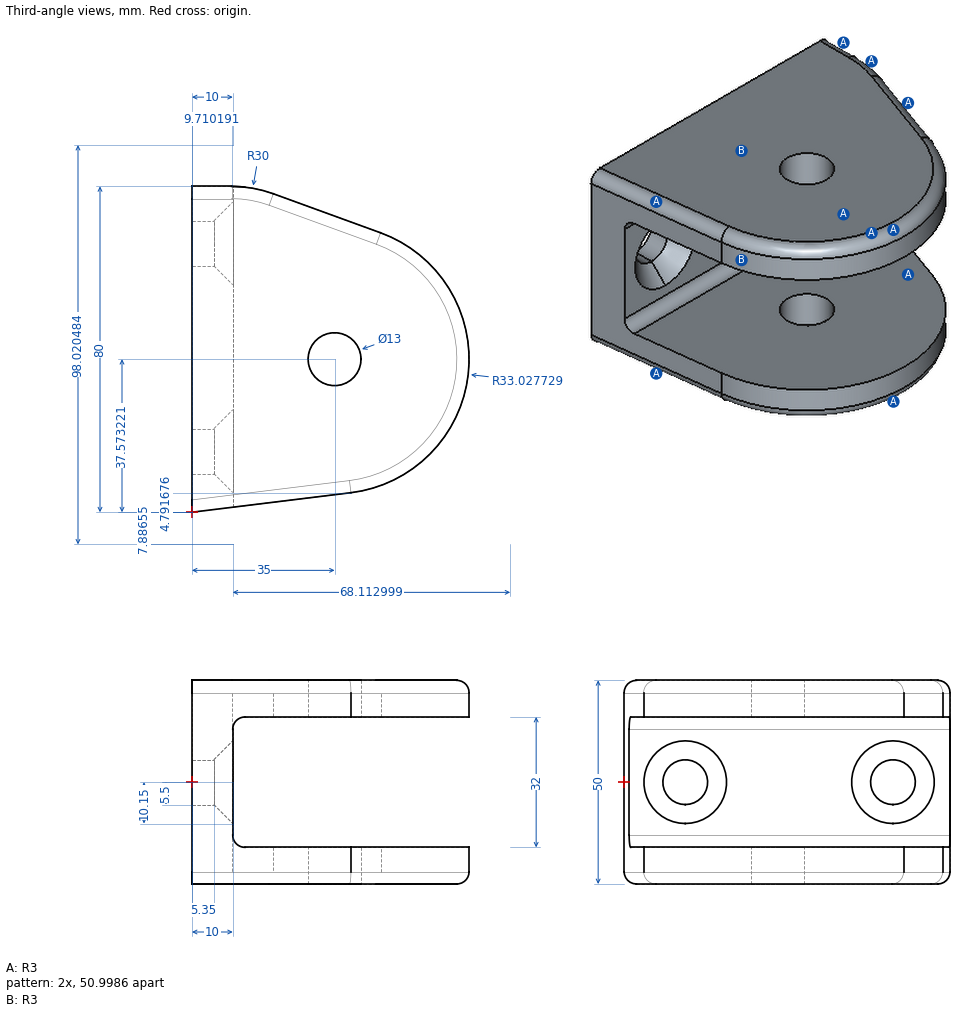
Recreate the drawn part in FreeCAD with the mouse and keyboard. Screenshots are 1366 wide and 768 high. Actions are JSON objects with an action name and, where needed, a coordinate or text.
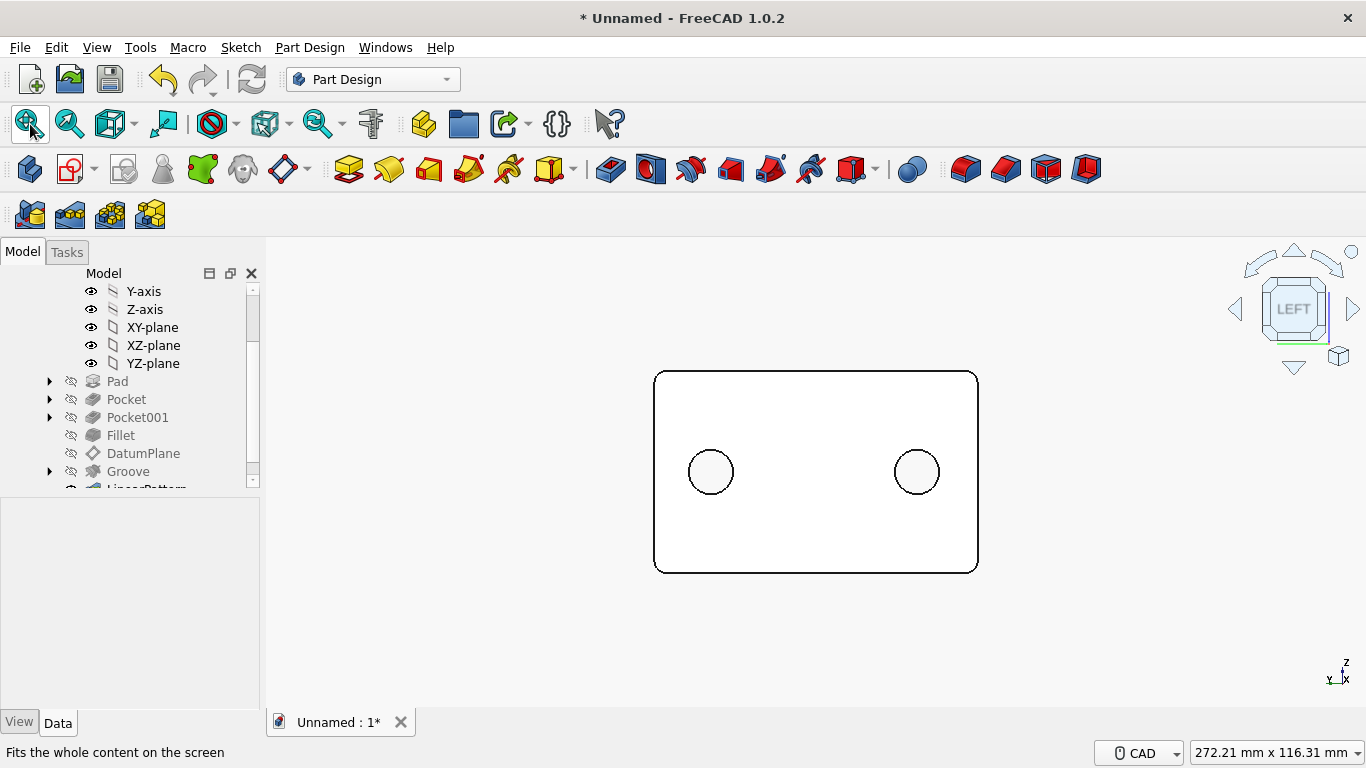
{"action": "key", "text": "v 3"}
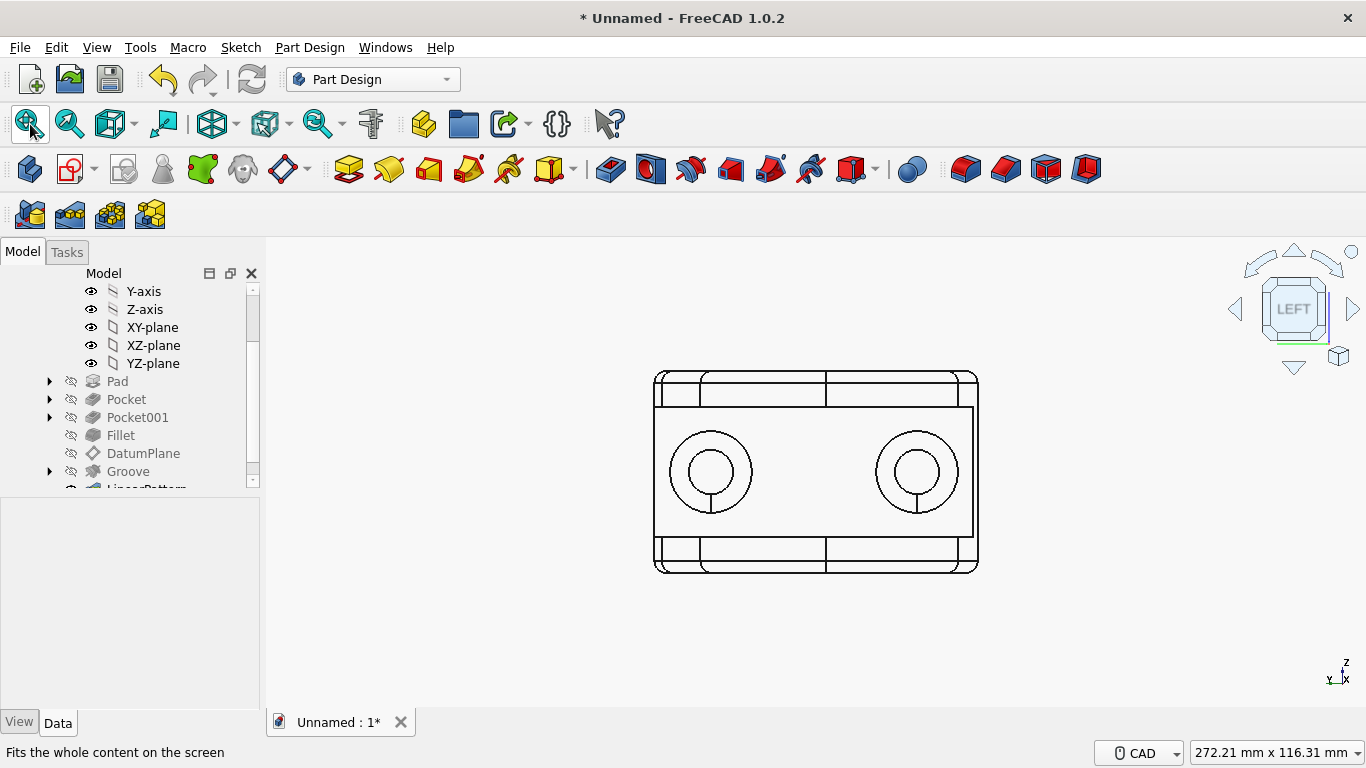
{"action": "key", "text": "0"}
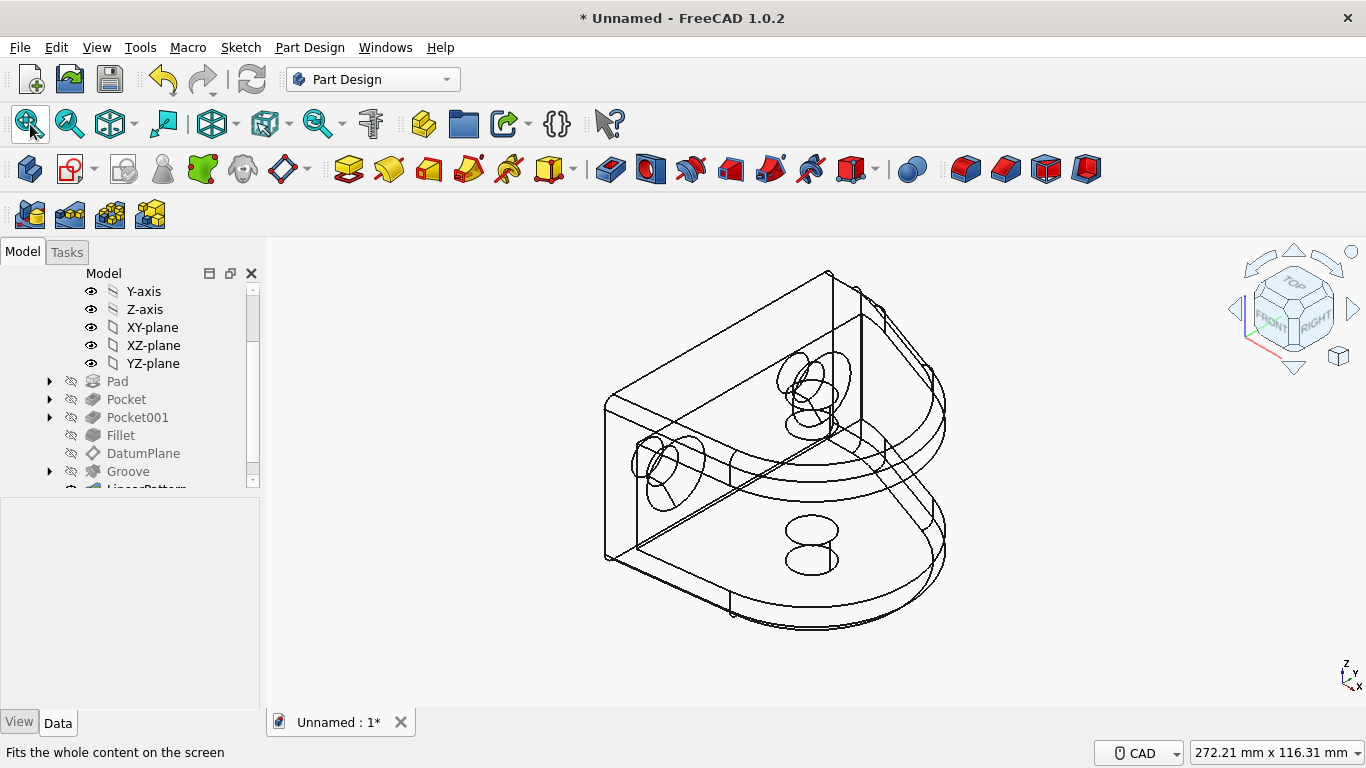
{"action": "left_click", "coordinate": [749, 483]}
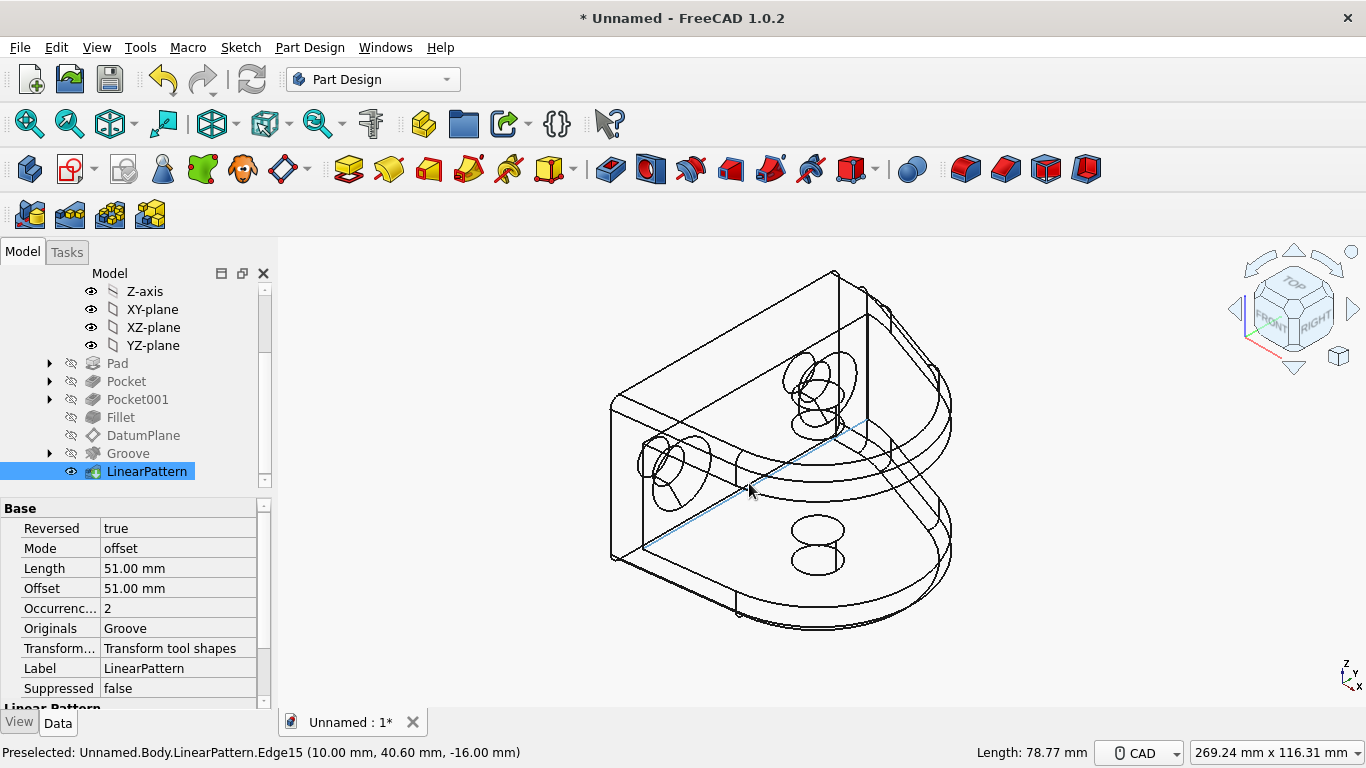
{"action": "left_click", "coordinate": [755, 378], "text": "ctrl"}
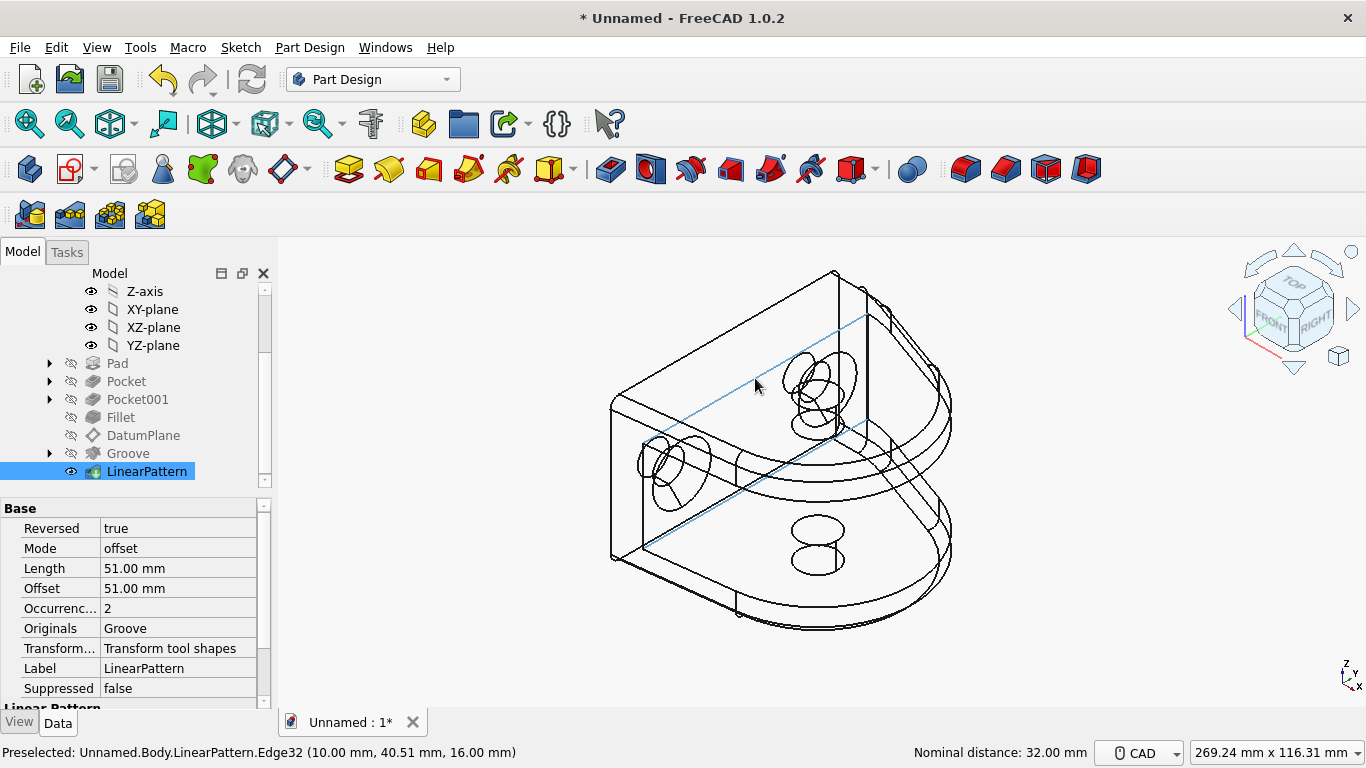
{"action": "key", "text": "v 1"}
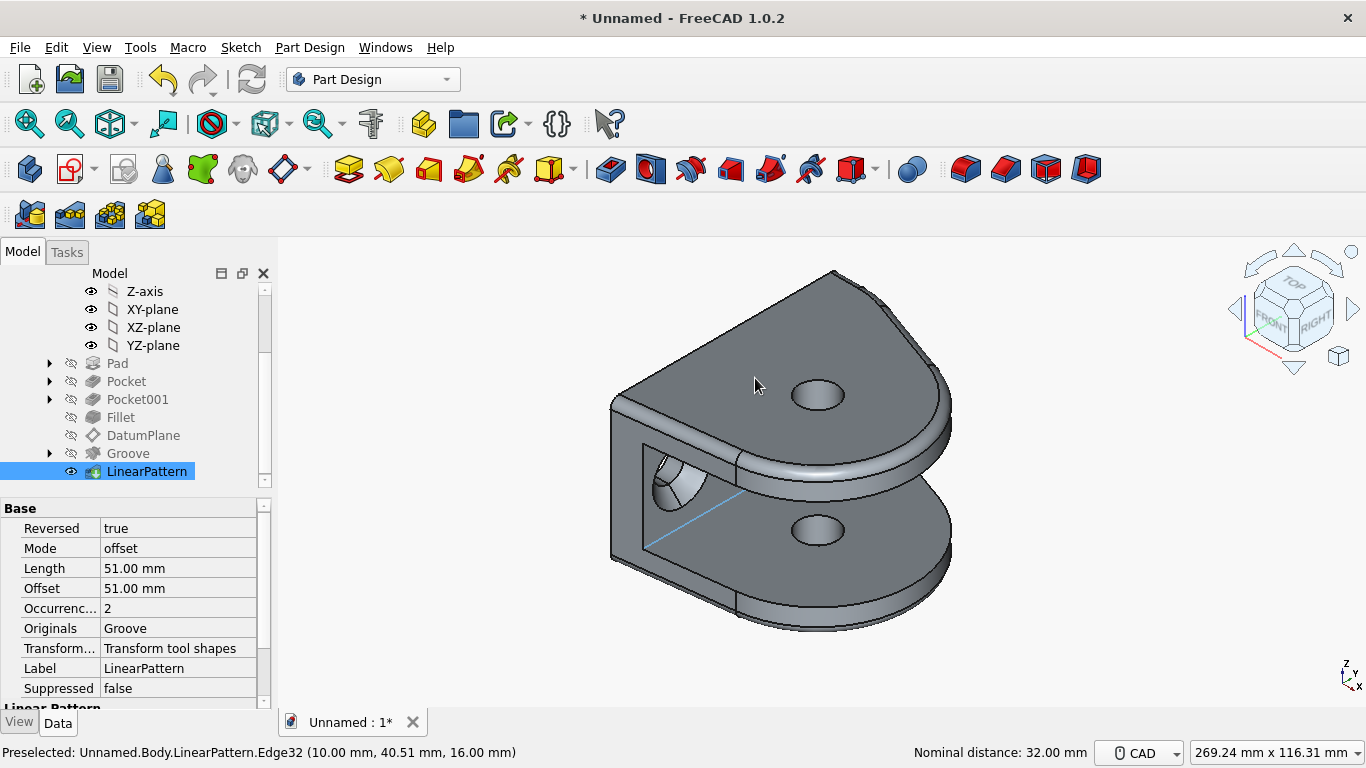
{"action": "left_click", "coordinate": [966, 170]}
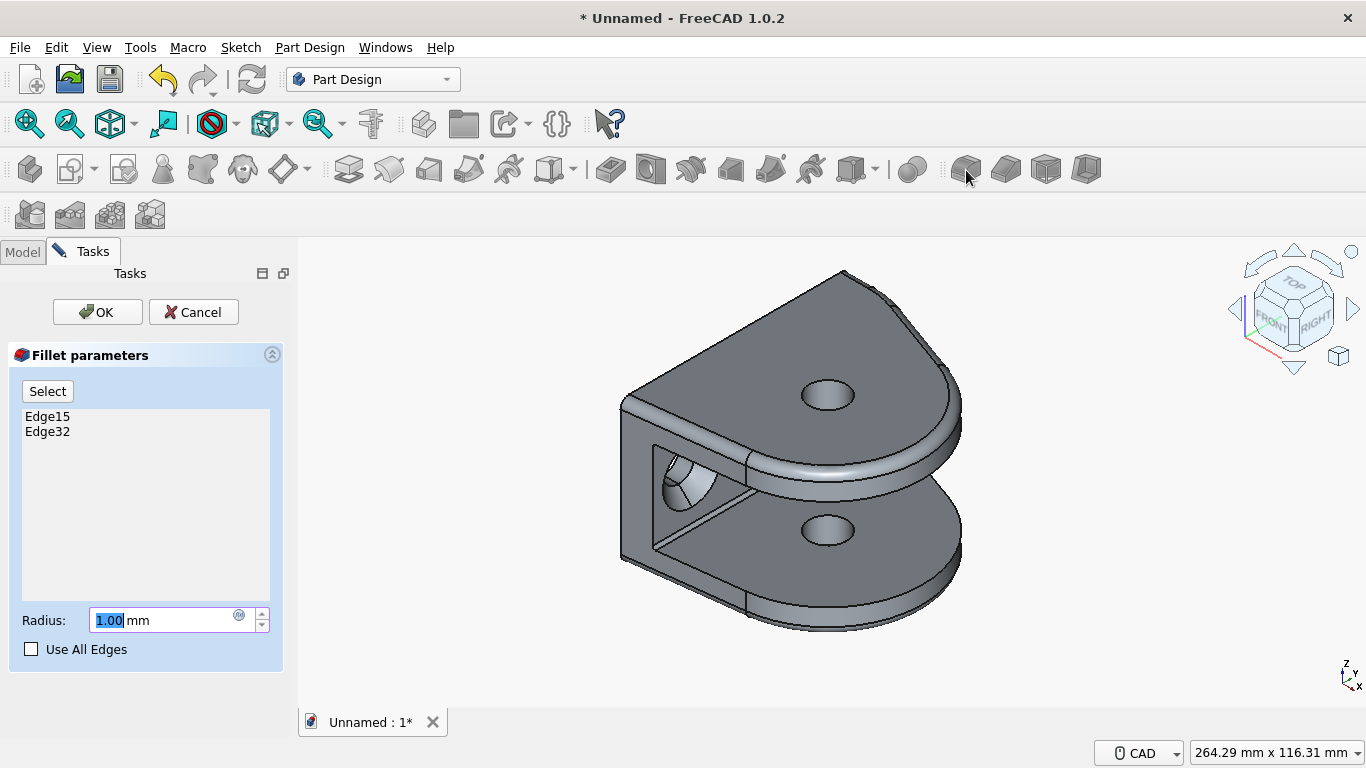
{"action": "type", "text": "3"}
{"action": "key", "text": "Tab"}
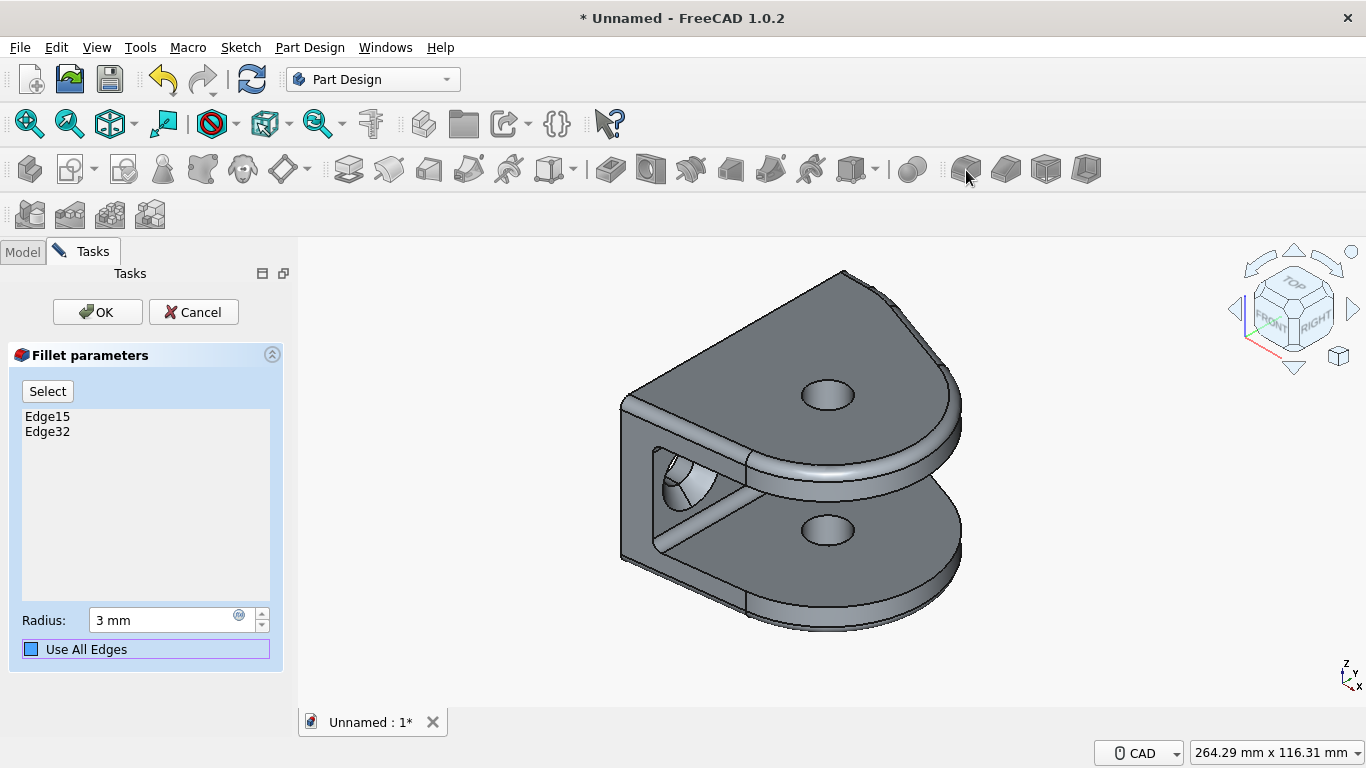
{"action": "left_click", "coordinate": [98, 312]}